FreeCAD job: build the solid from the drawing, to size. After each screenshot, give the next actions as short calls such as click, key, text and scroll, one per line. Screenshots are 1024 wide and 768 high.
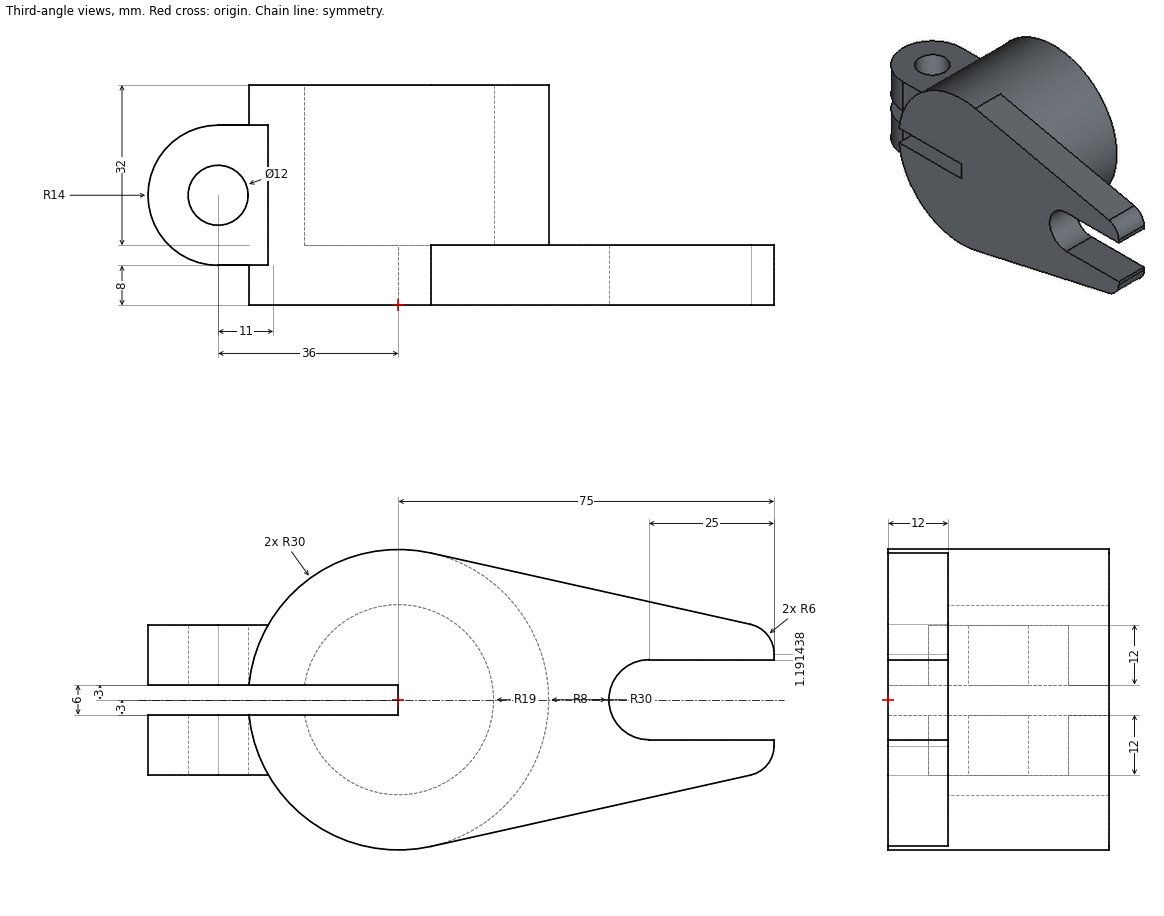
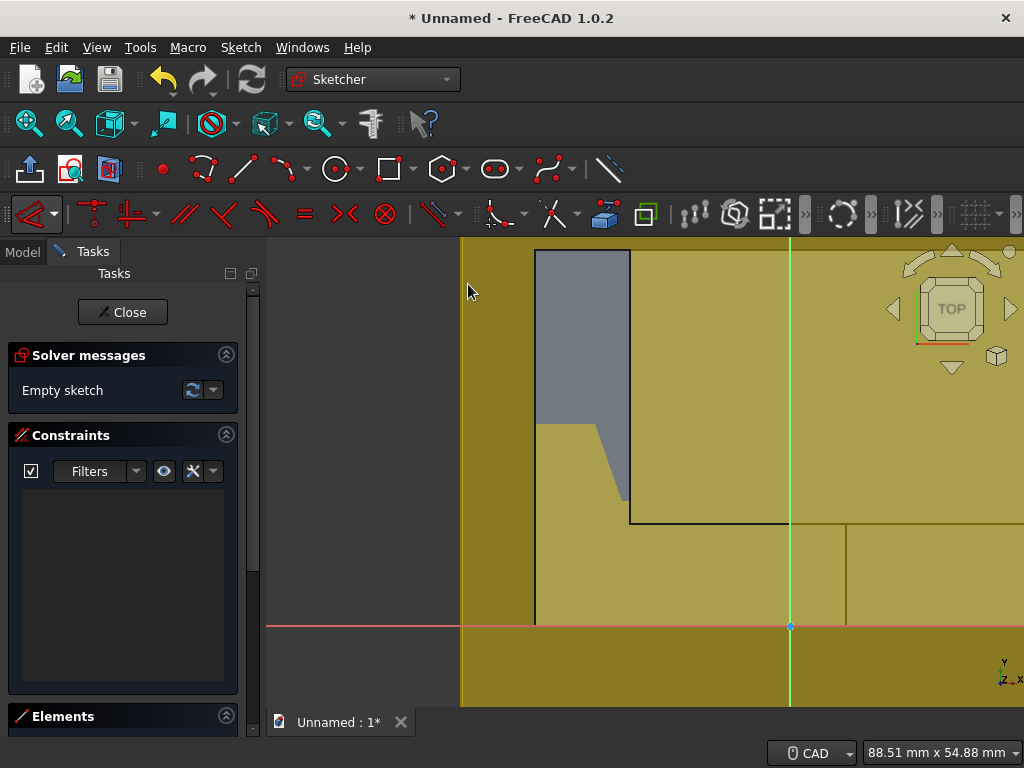
key(g)
key(m)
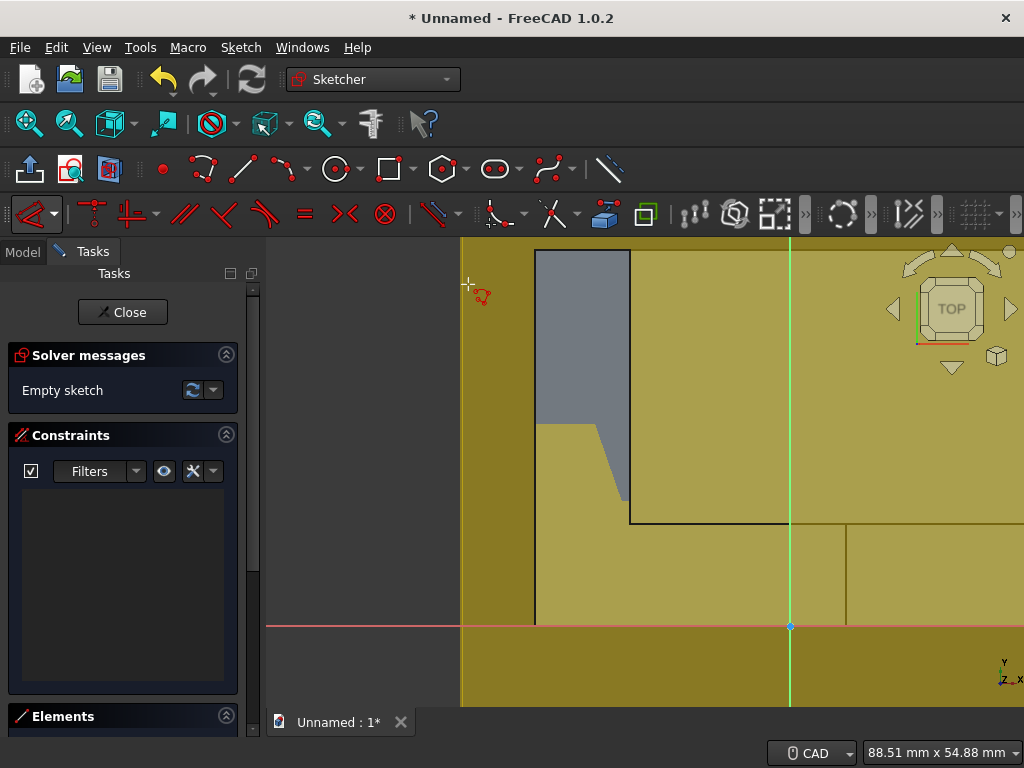
click(482, 558)
click(576, 558)
click(576, 318)
click(482, 318)
right_click(482, 318)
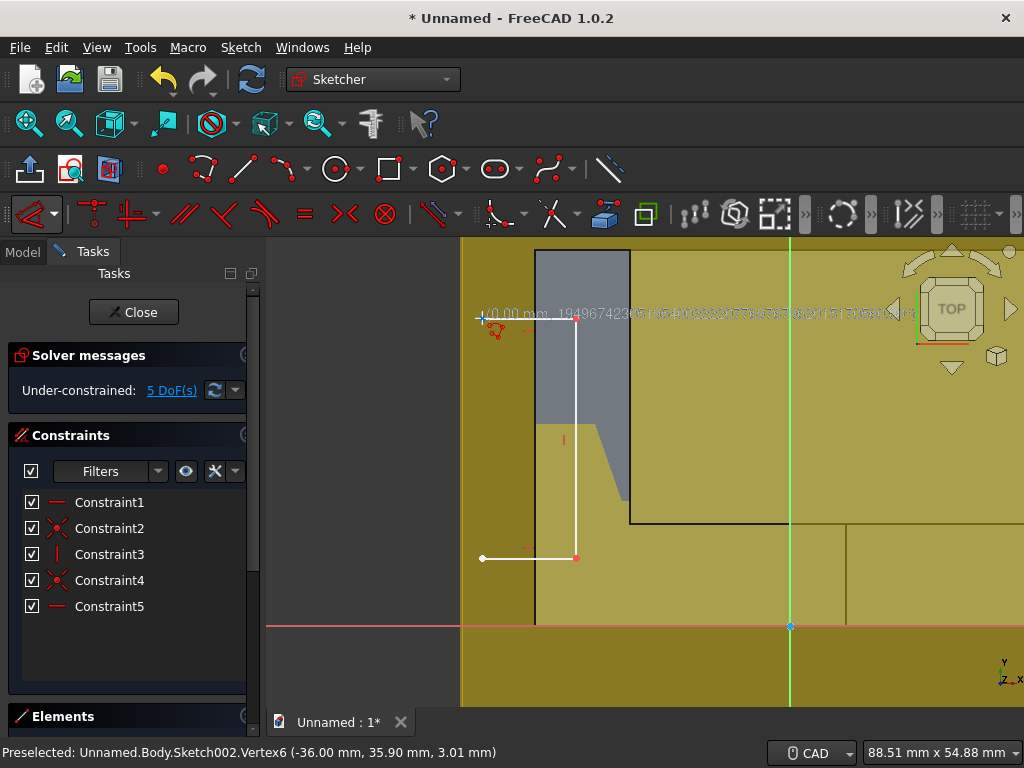
key(g)
key(3)
key(a)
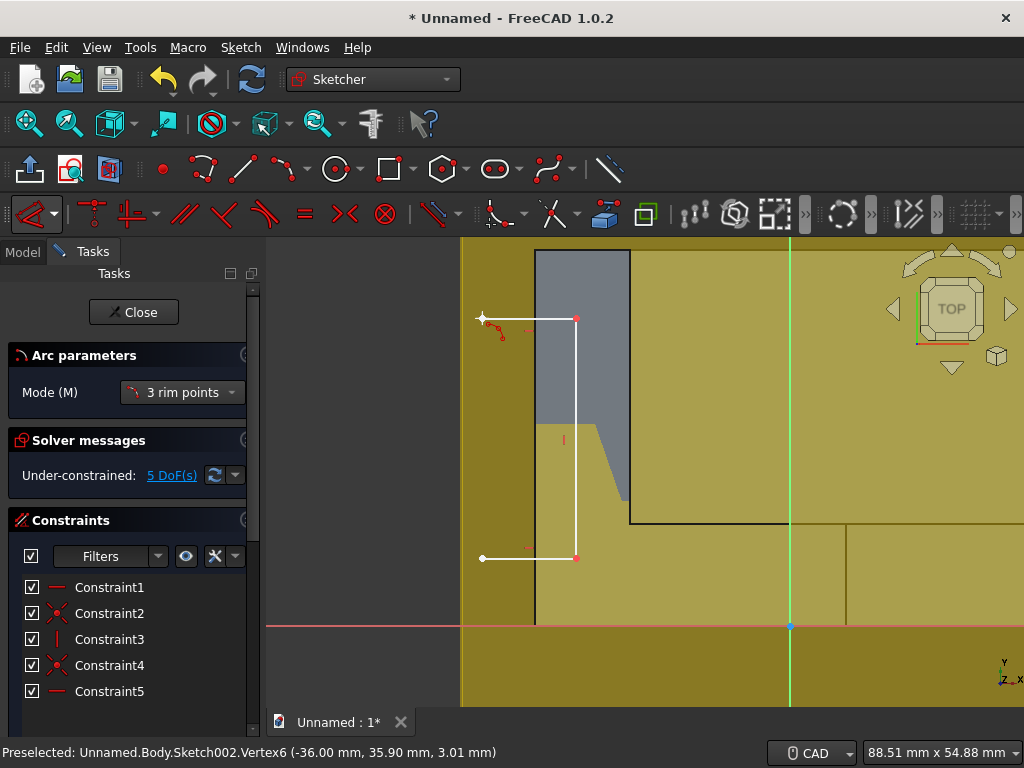
click(482, 319)
click(482, 559)
click(362, 438)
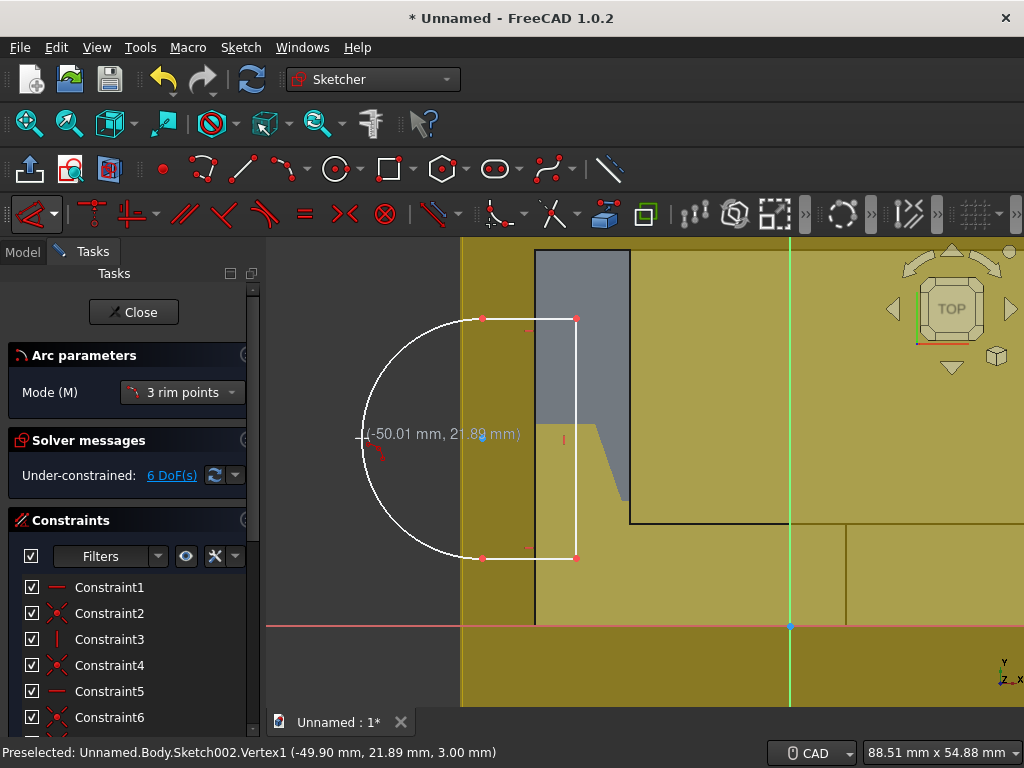
click(336, 170)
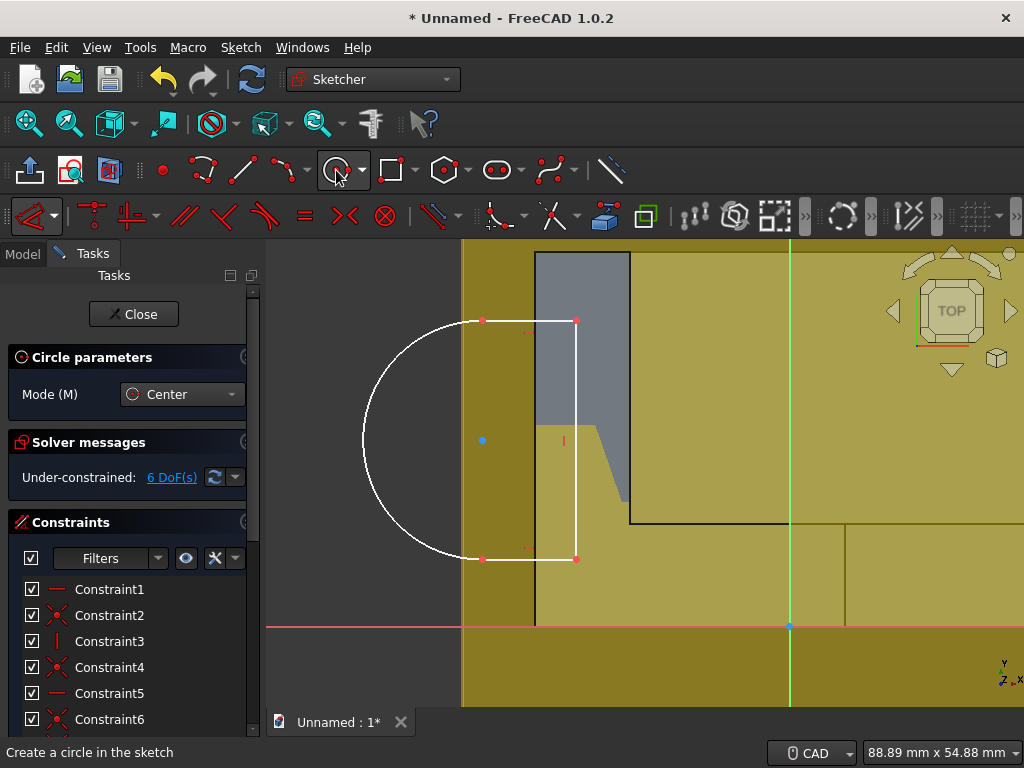
click(483, 439)
click(519, 403)
key(Escape)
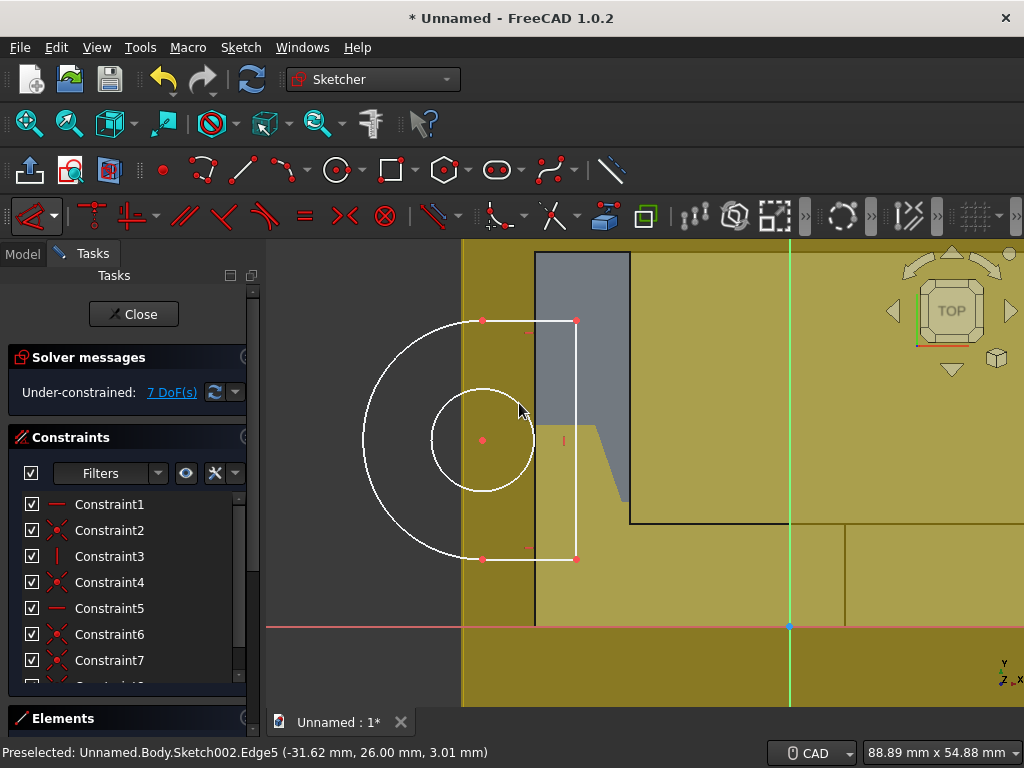
click(511, 560)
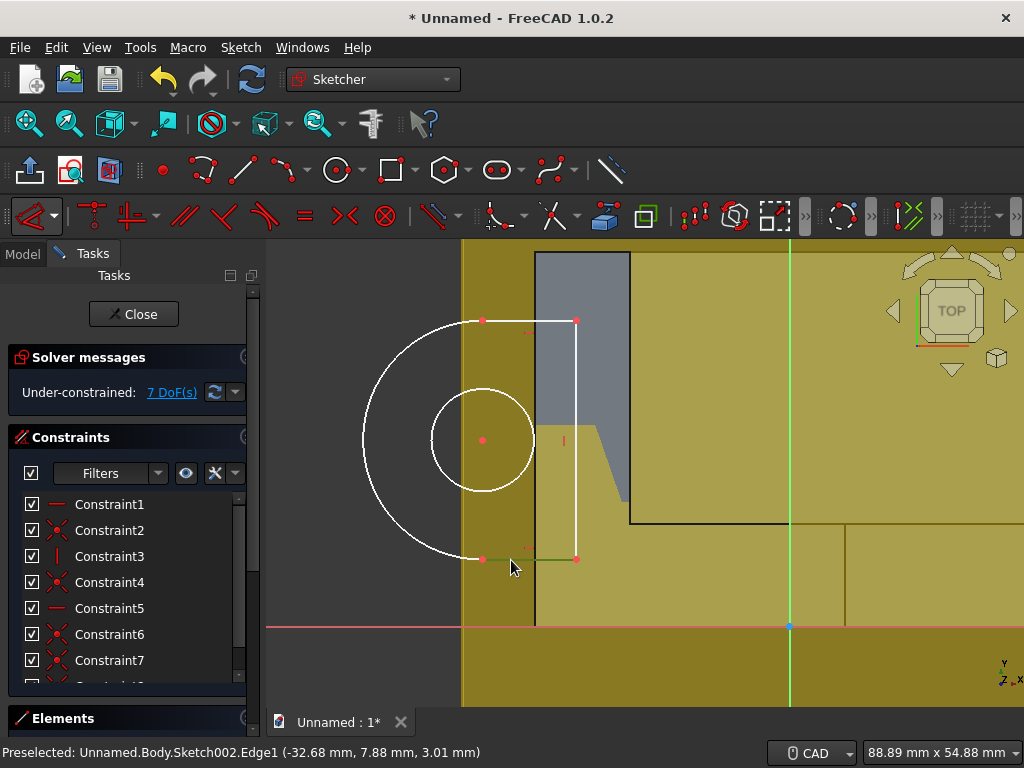
click(386, 370)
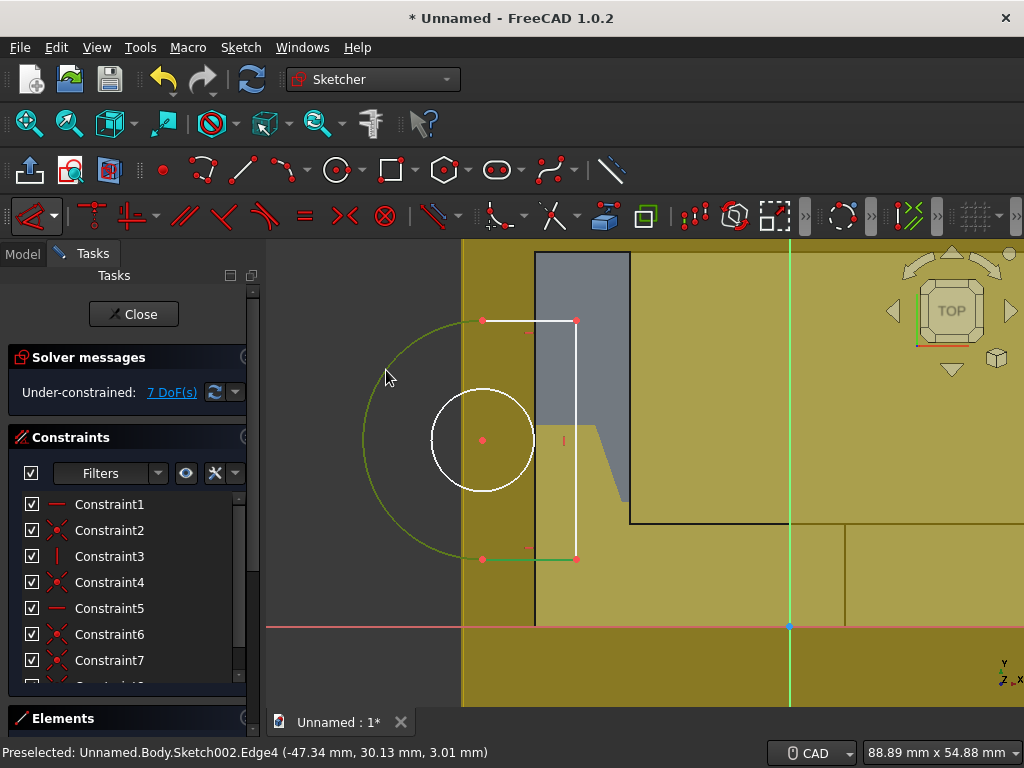
key(t)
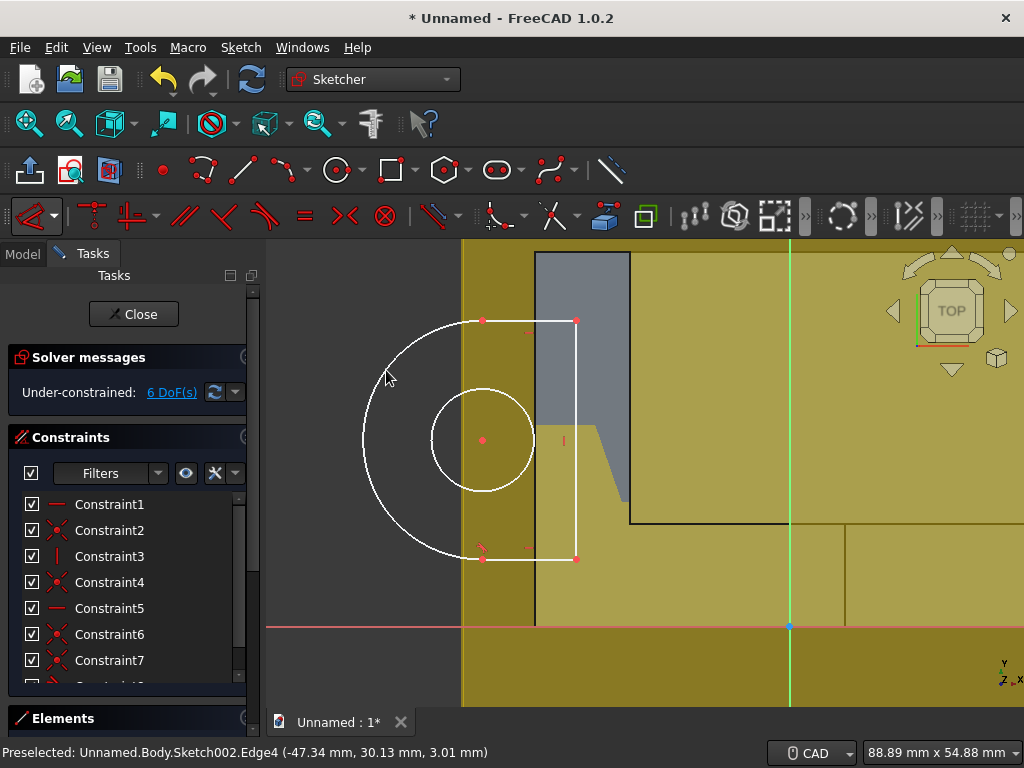
click(548, 321)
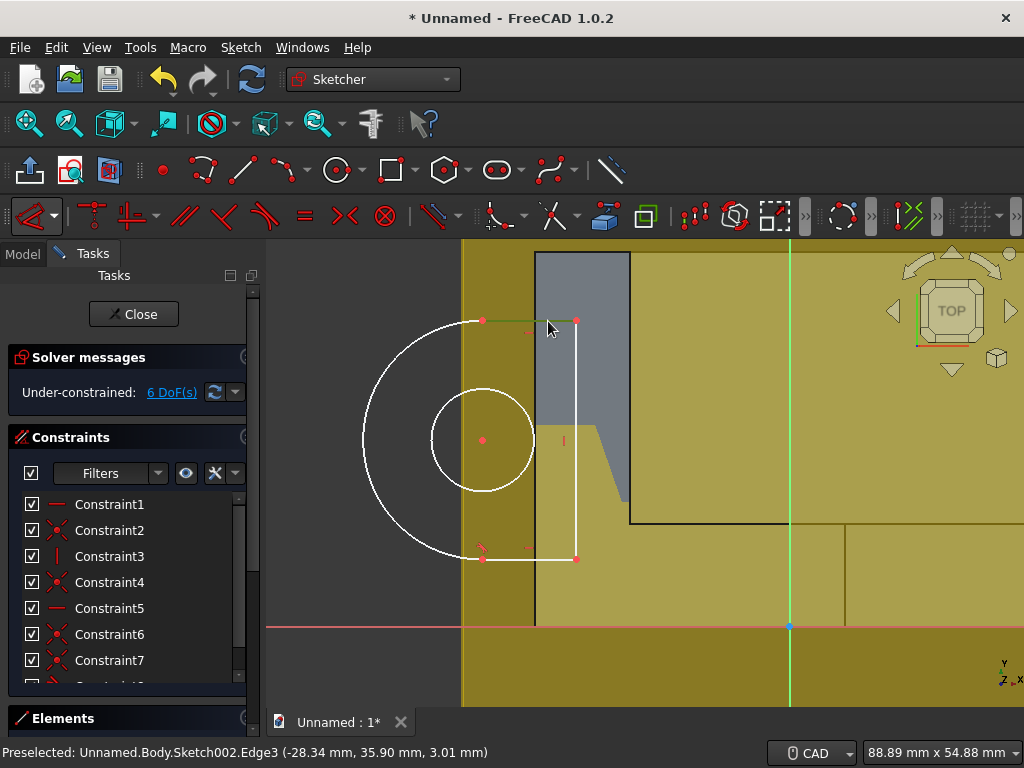
click(386, 370)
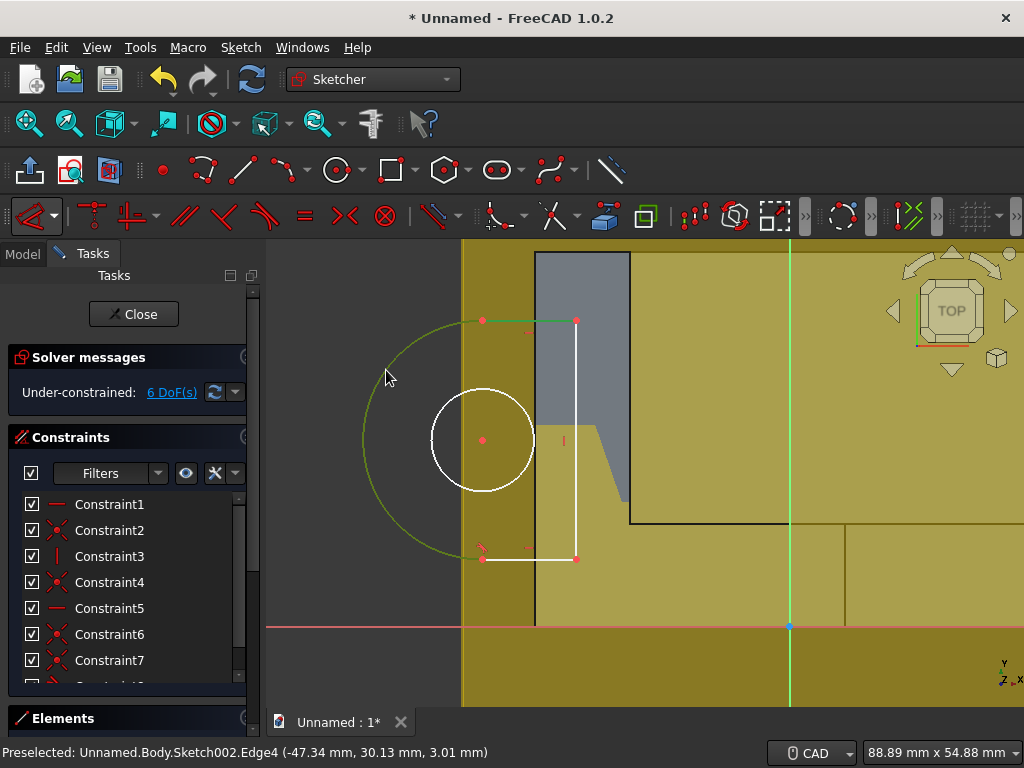
click(266, 216)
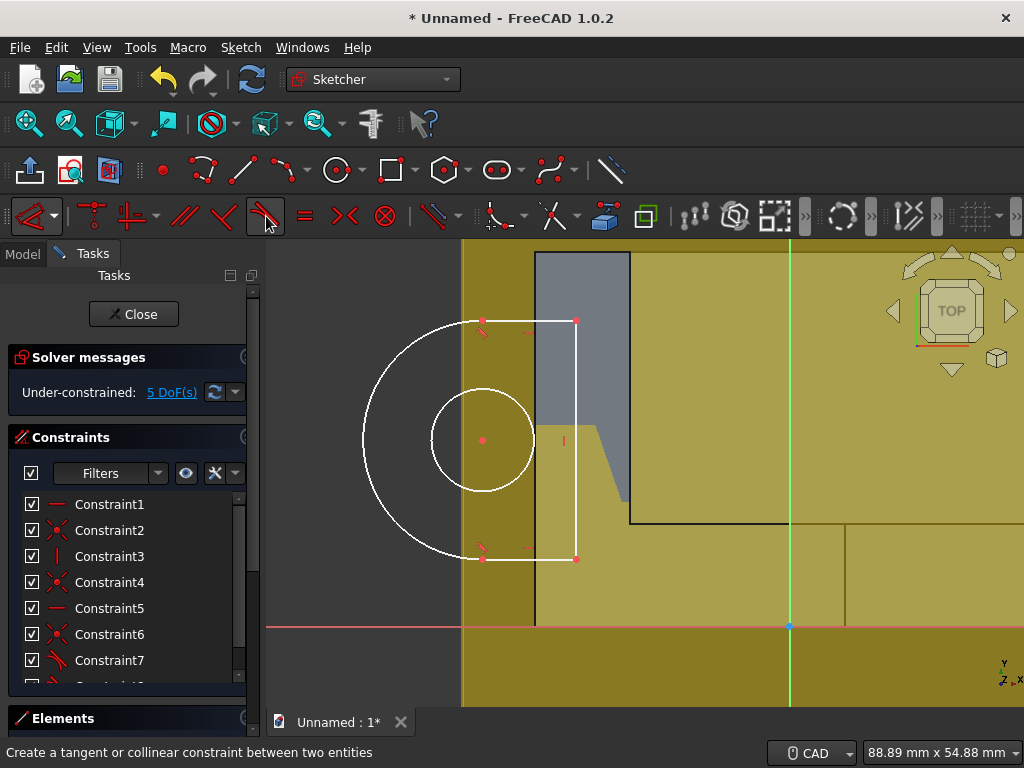
click(386, 370)